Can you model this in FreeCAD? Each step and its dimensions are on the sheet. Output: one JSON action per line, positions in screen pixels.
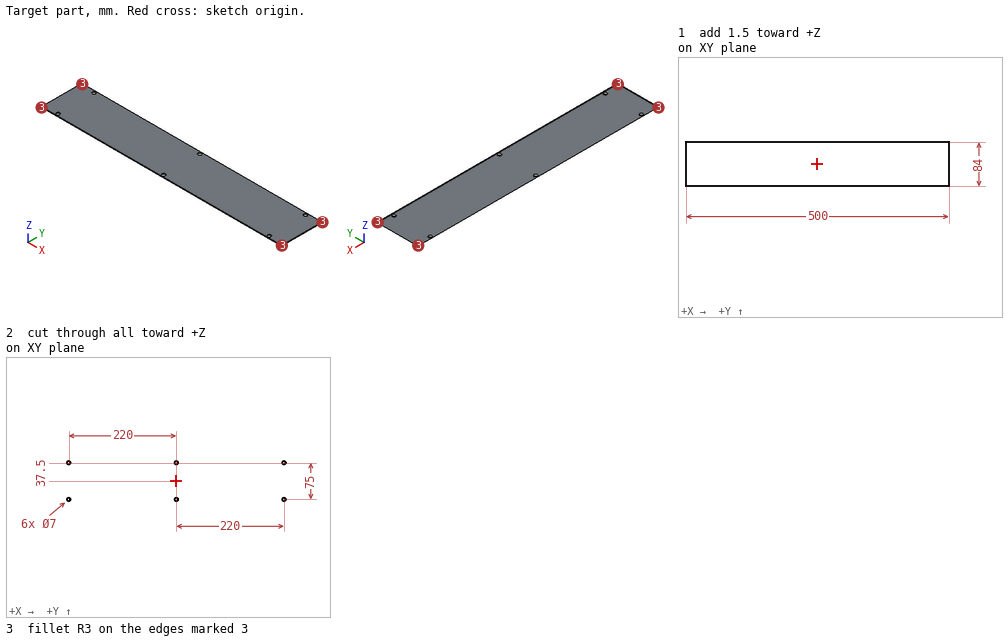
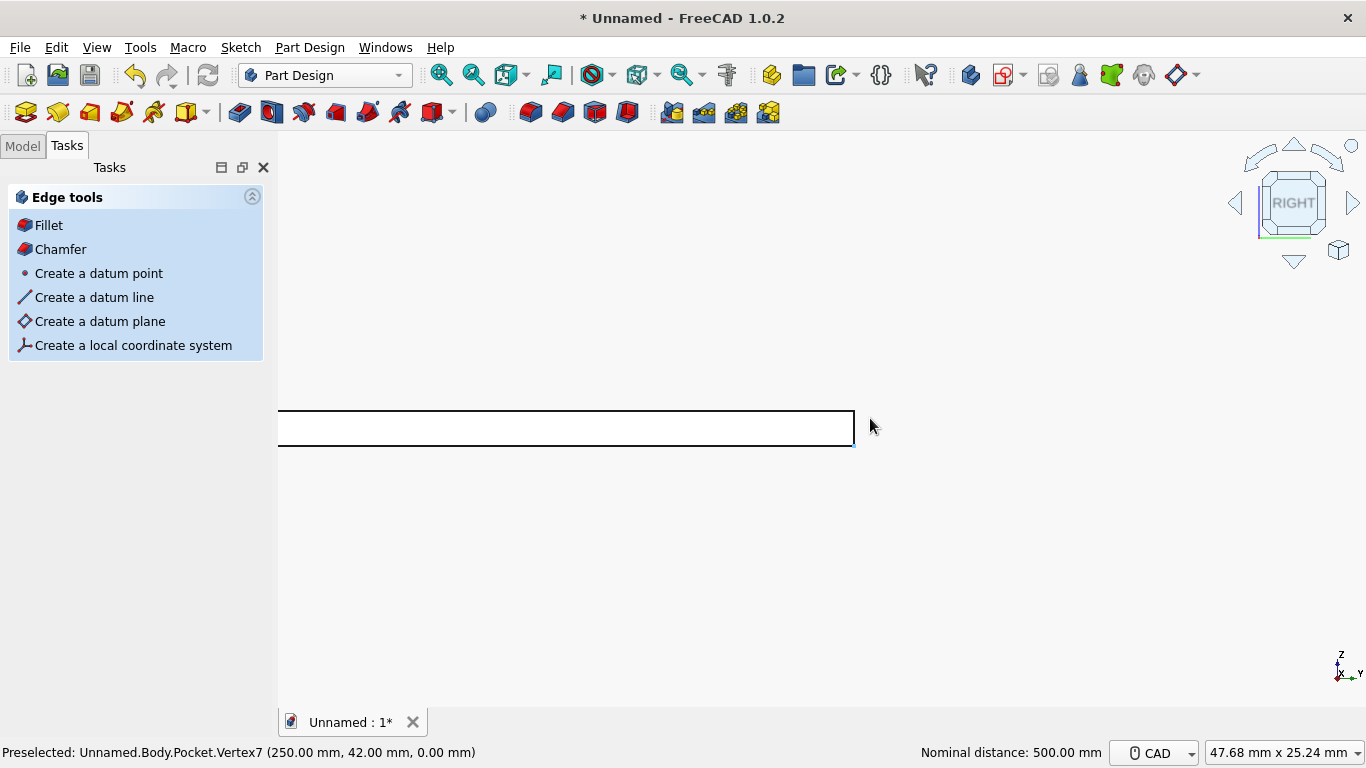
{"action": "left_click", "coordinate": [854, 428], "text": "ctrl"}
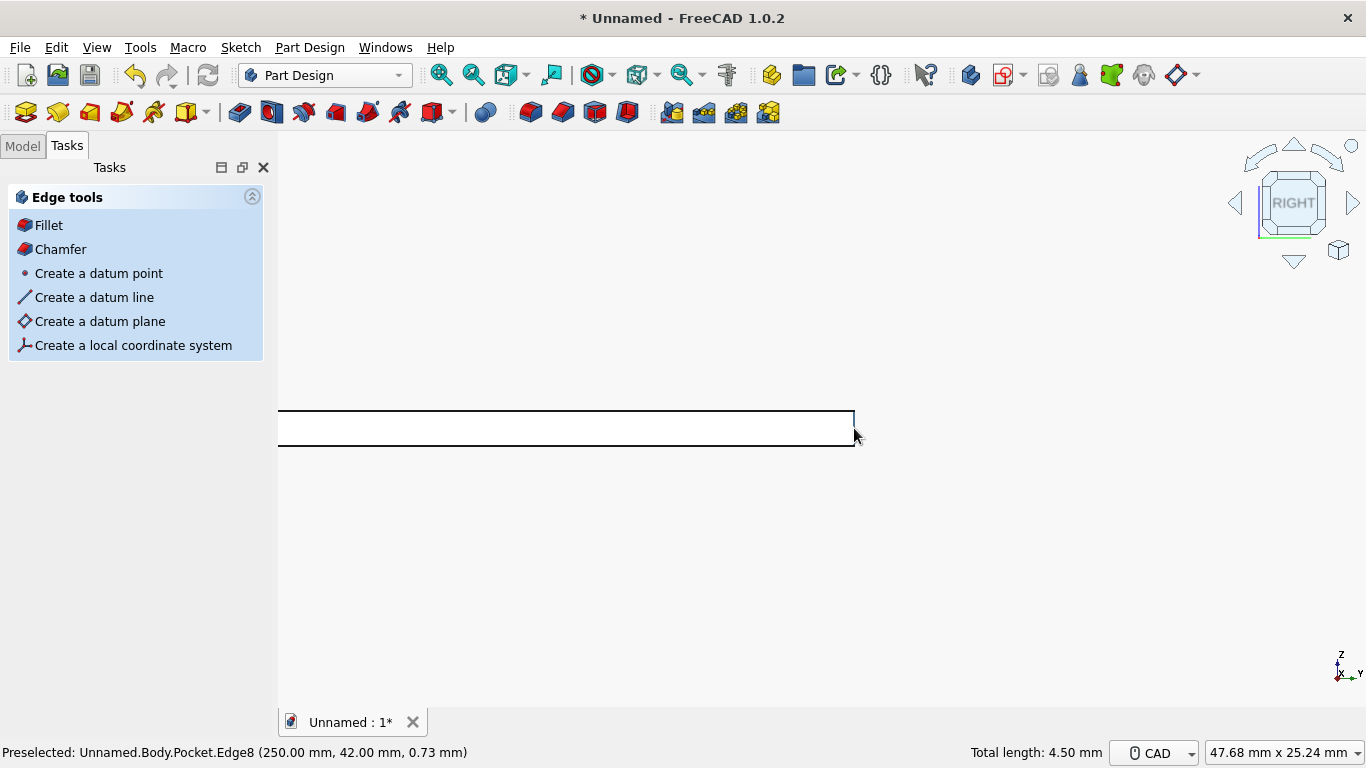
{"action": "left_click", "coordinate": [442, 76]}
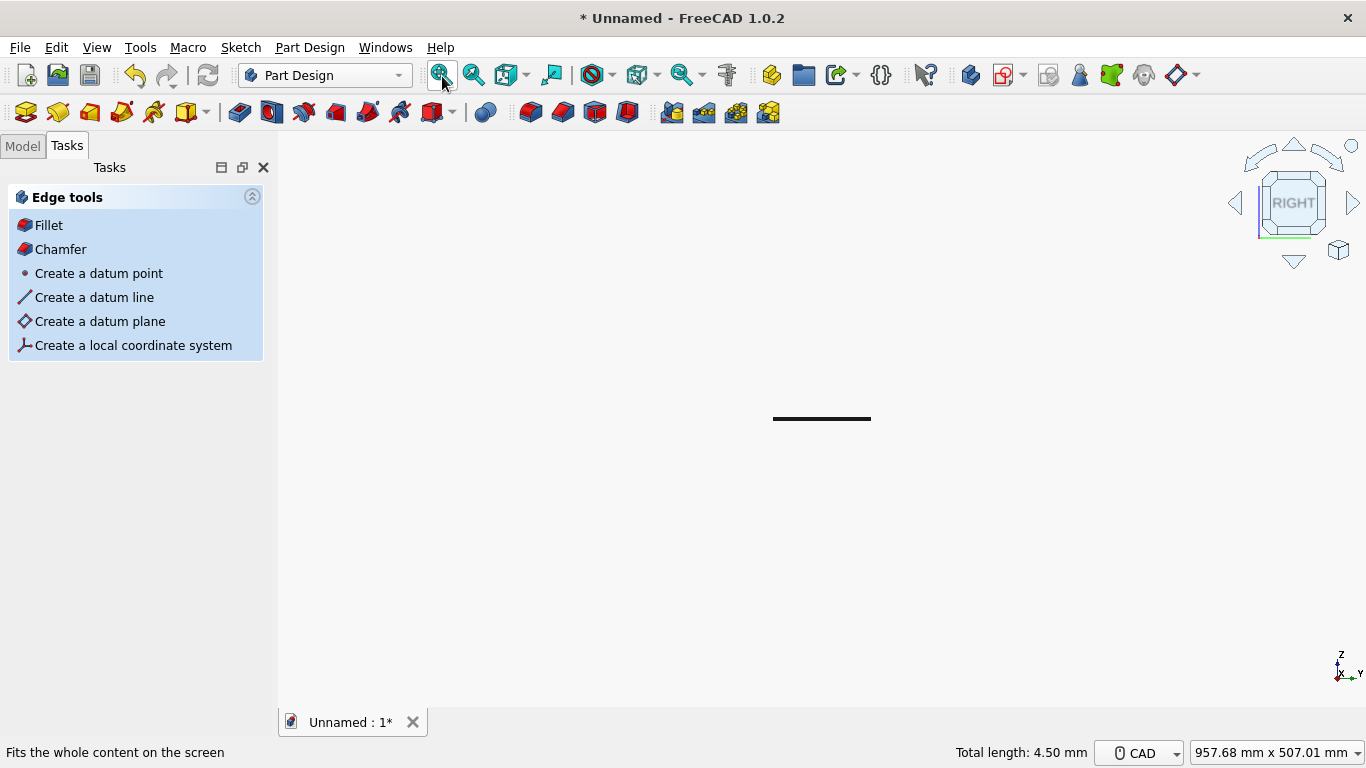
{"action": "key", "text": "5"}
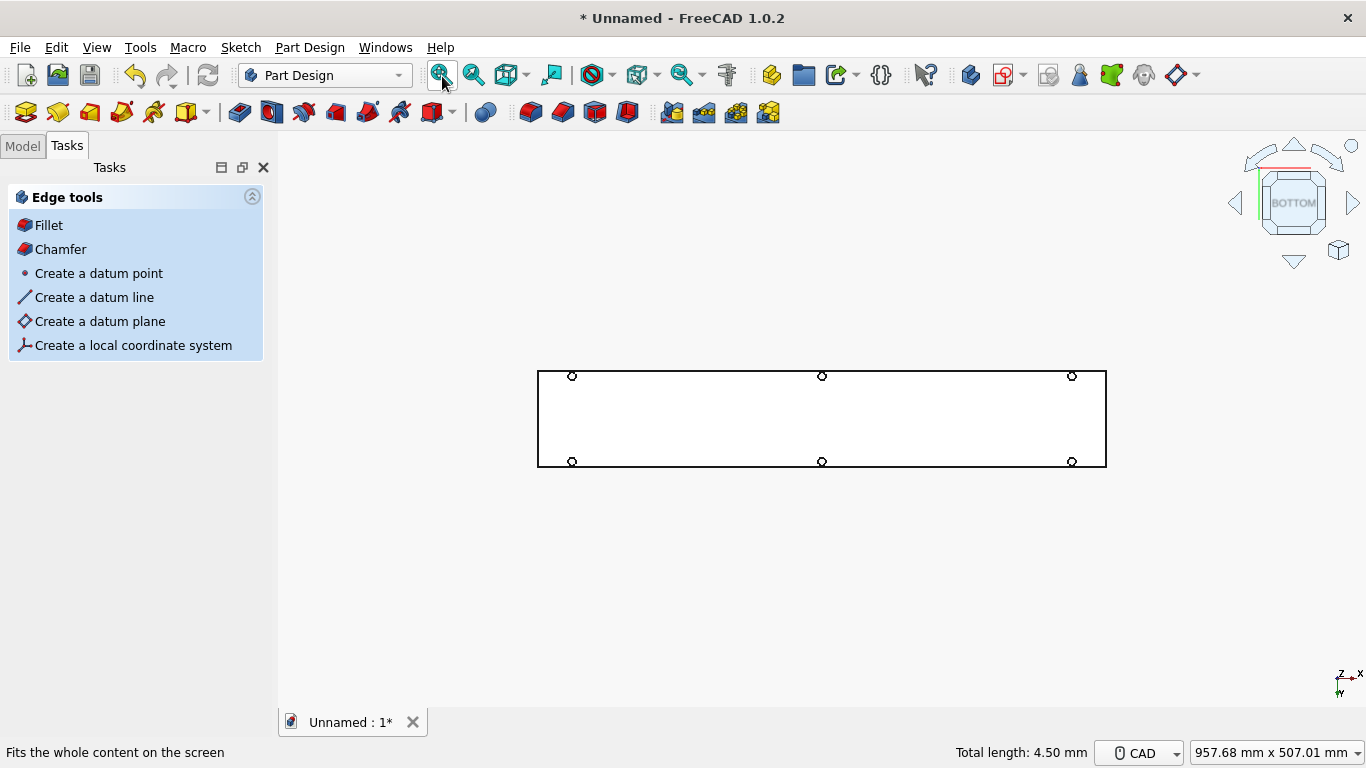
{"action": "scroll", "coordinate": [538, 466], "scroll_direction": "up", "scroll_amount": 15}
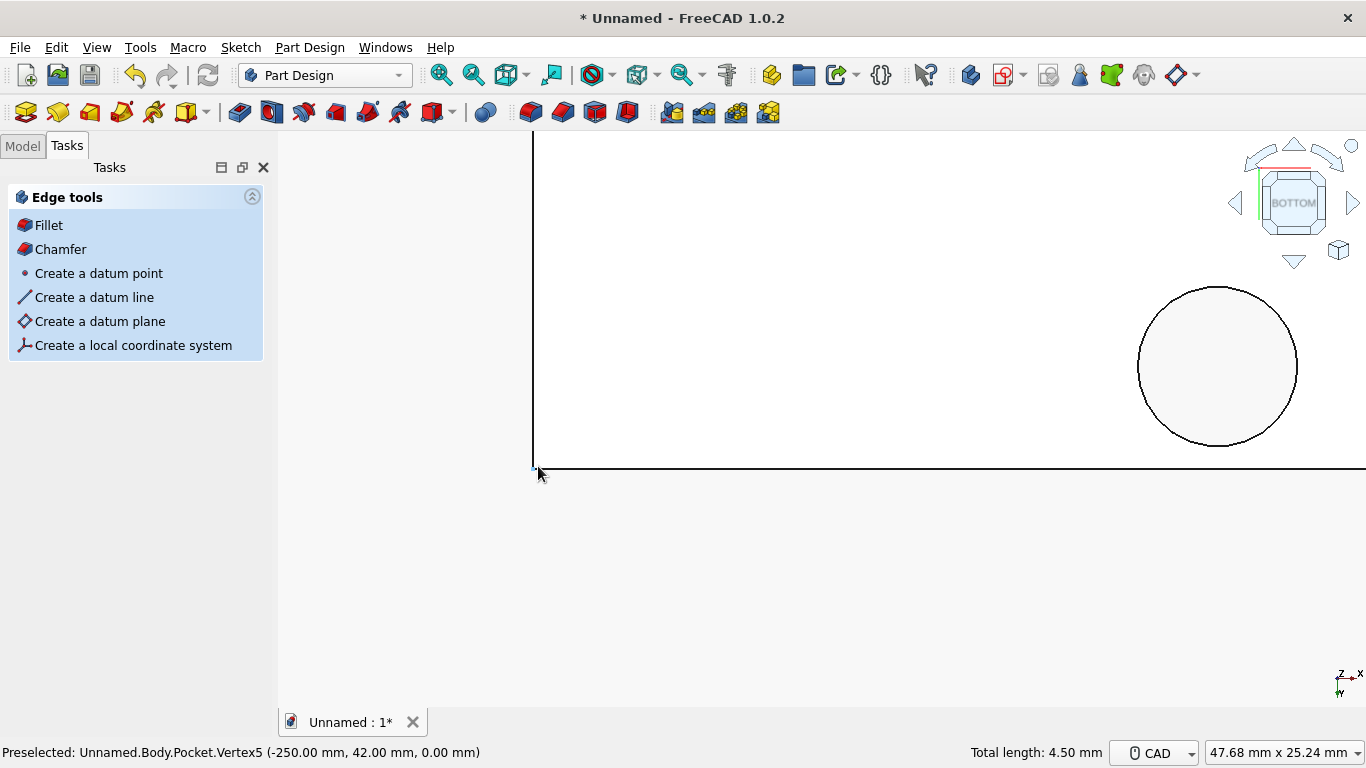
{"action": "left_click", "coordinate": [442, 76]}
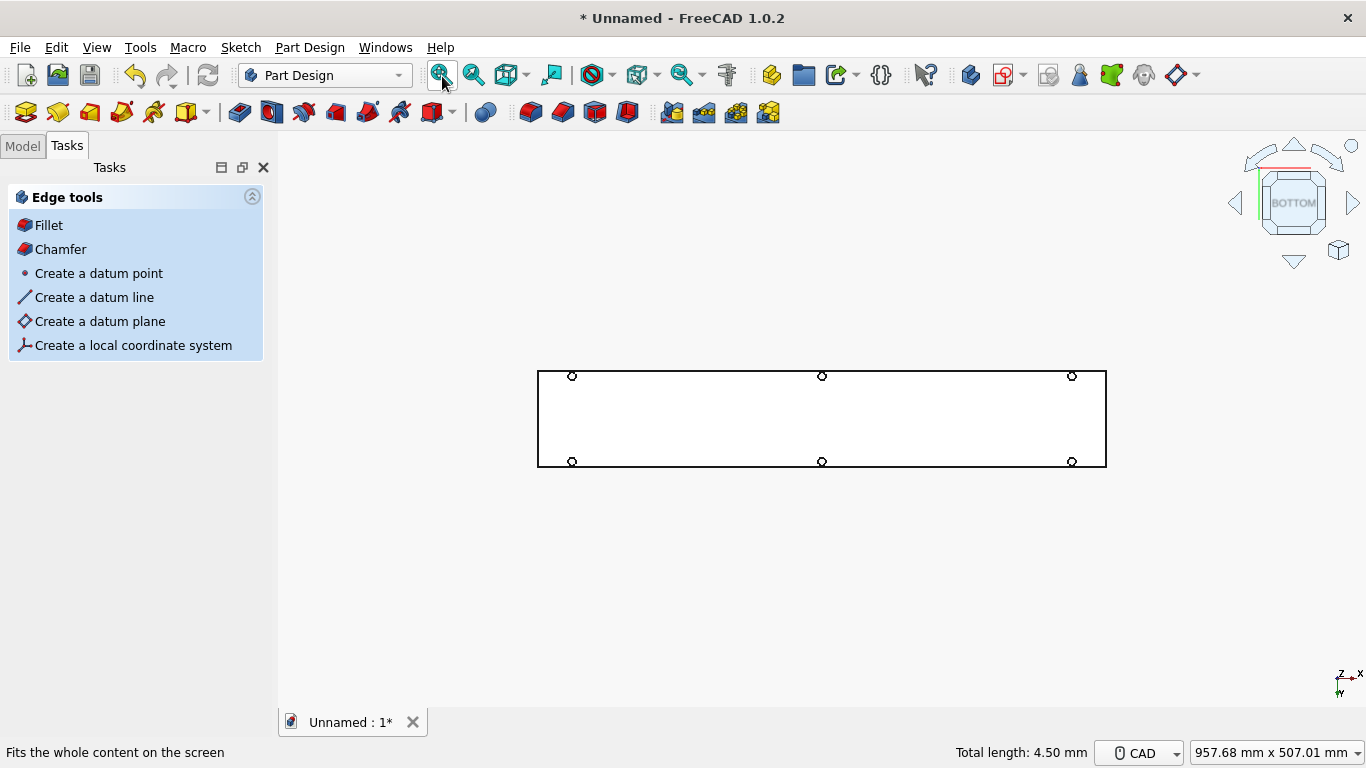
{"action": "key", "text": "4"}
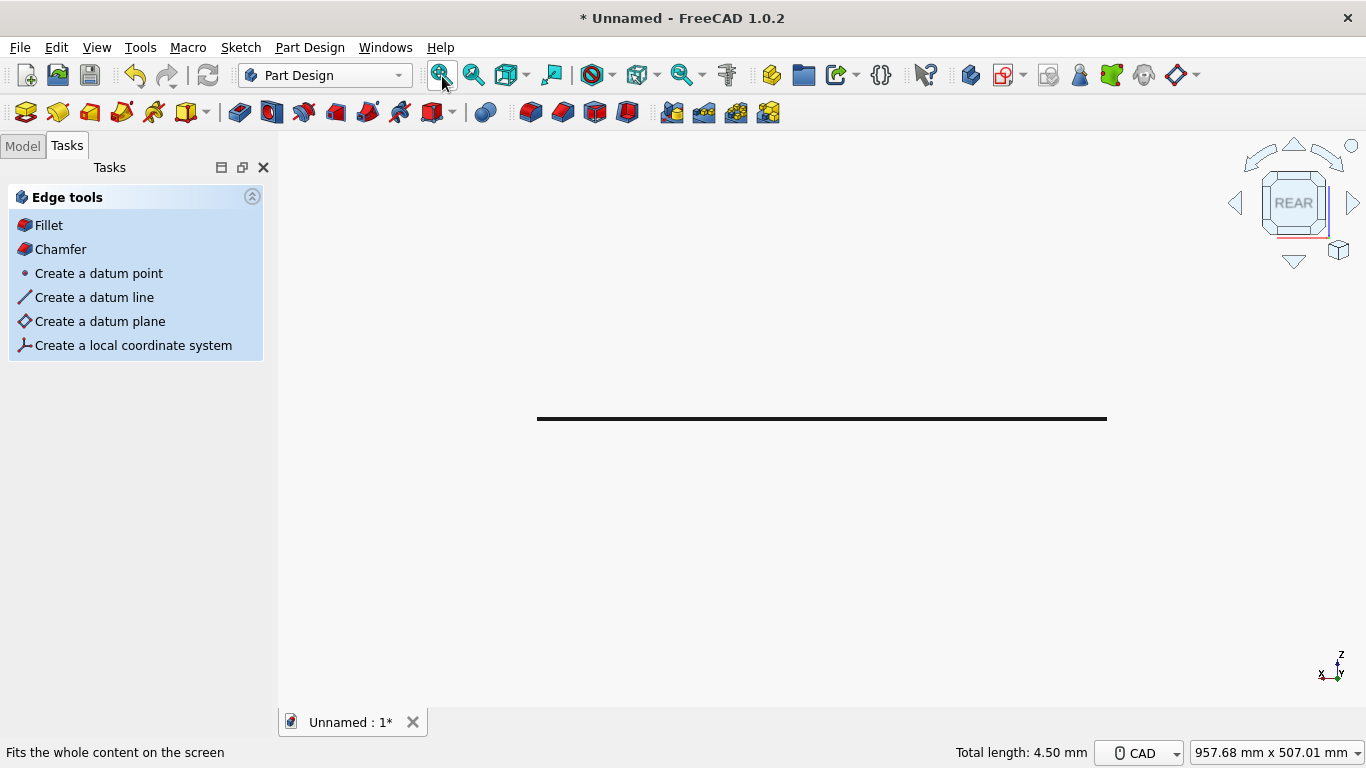
{"action": "scroll", "coordinate": [1106, 418], "scroll_direction": "up", "scroll_amount": 15}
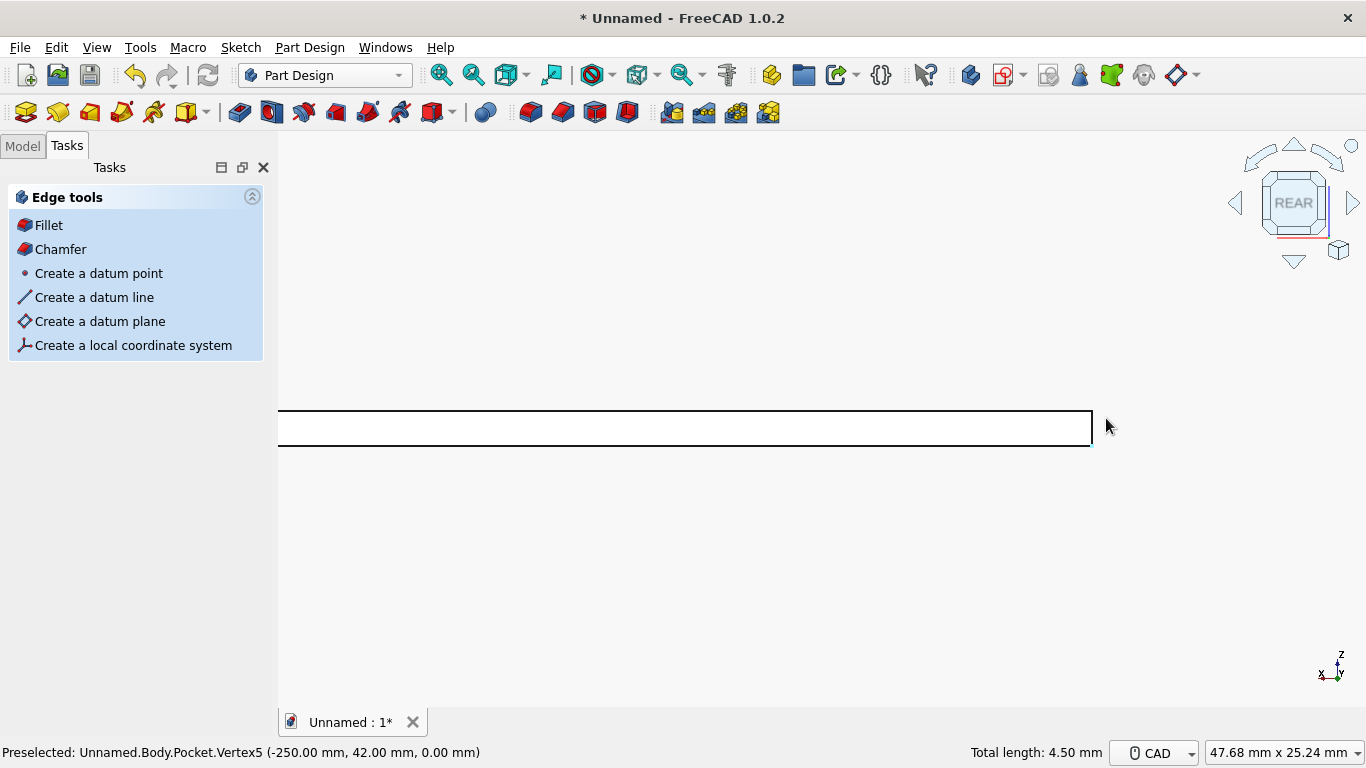
{"action": "left_click", "coordinate": [1092, 428], "text": "ctrl"}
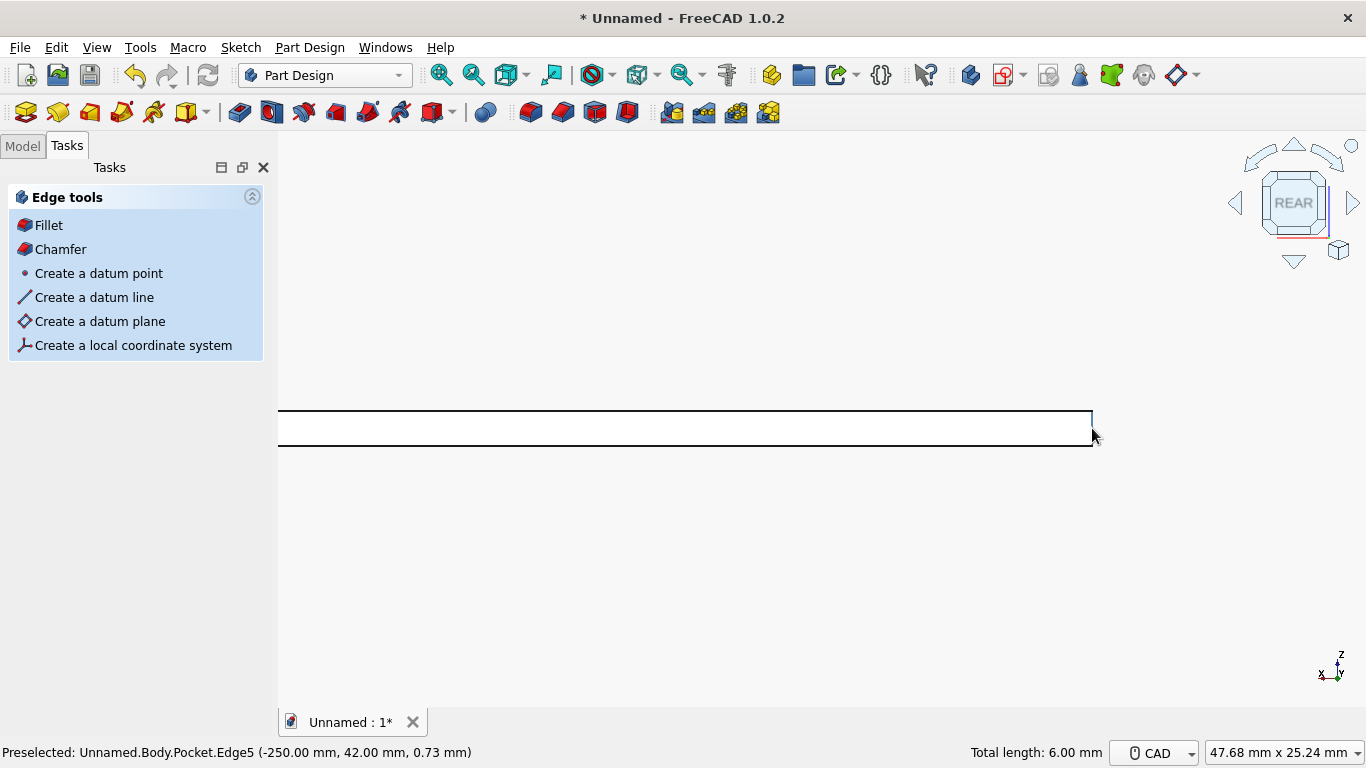
{"action": "left_click", "coordinate": [532, 112]}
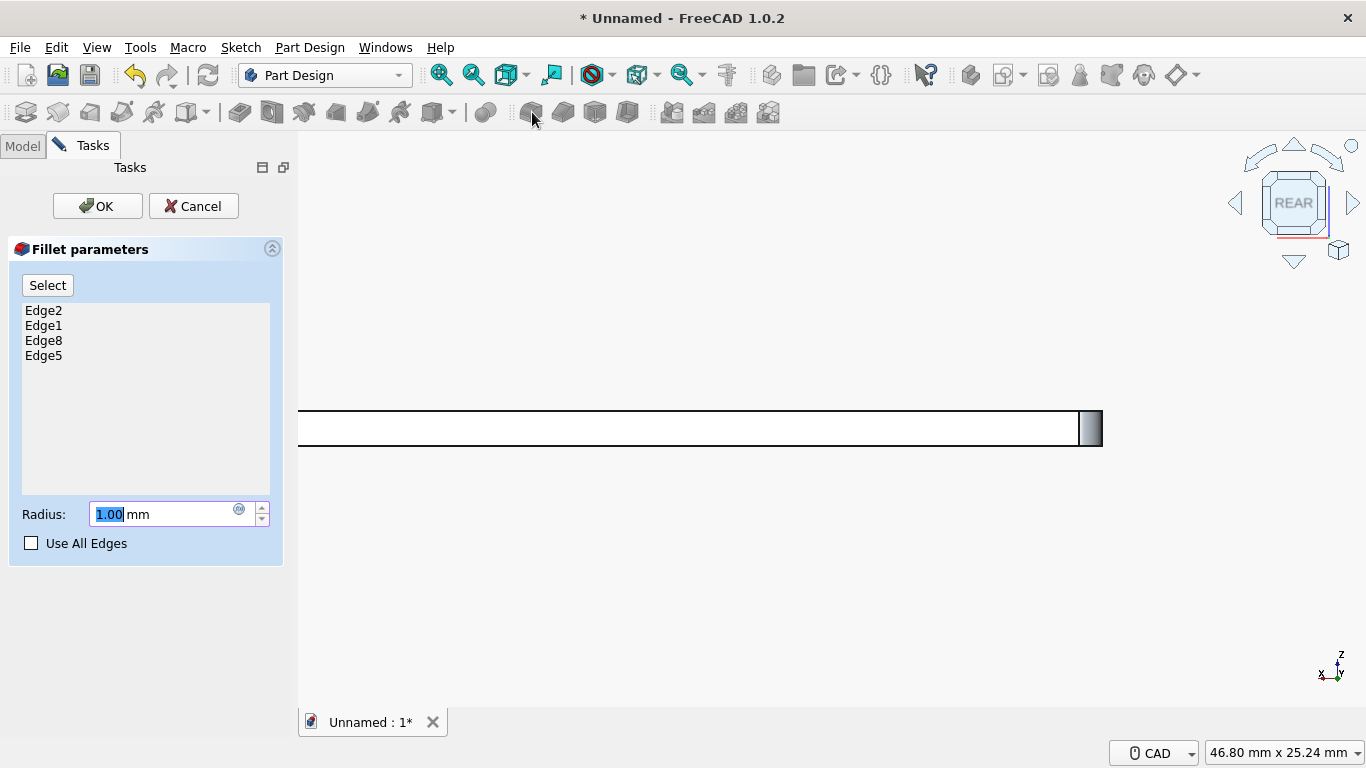
{"action": "type", "text": "3"}
{"action": "key", "text": "Tab"}